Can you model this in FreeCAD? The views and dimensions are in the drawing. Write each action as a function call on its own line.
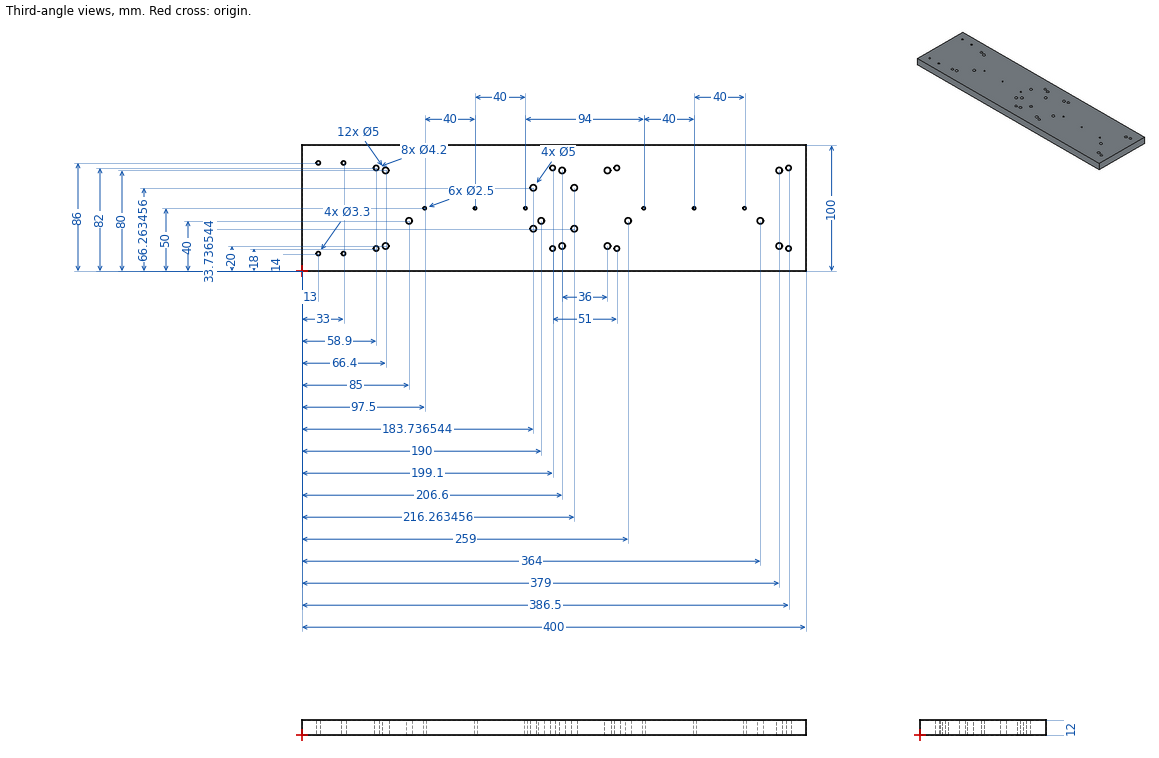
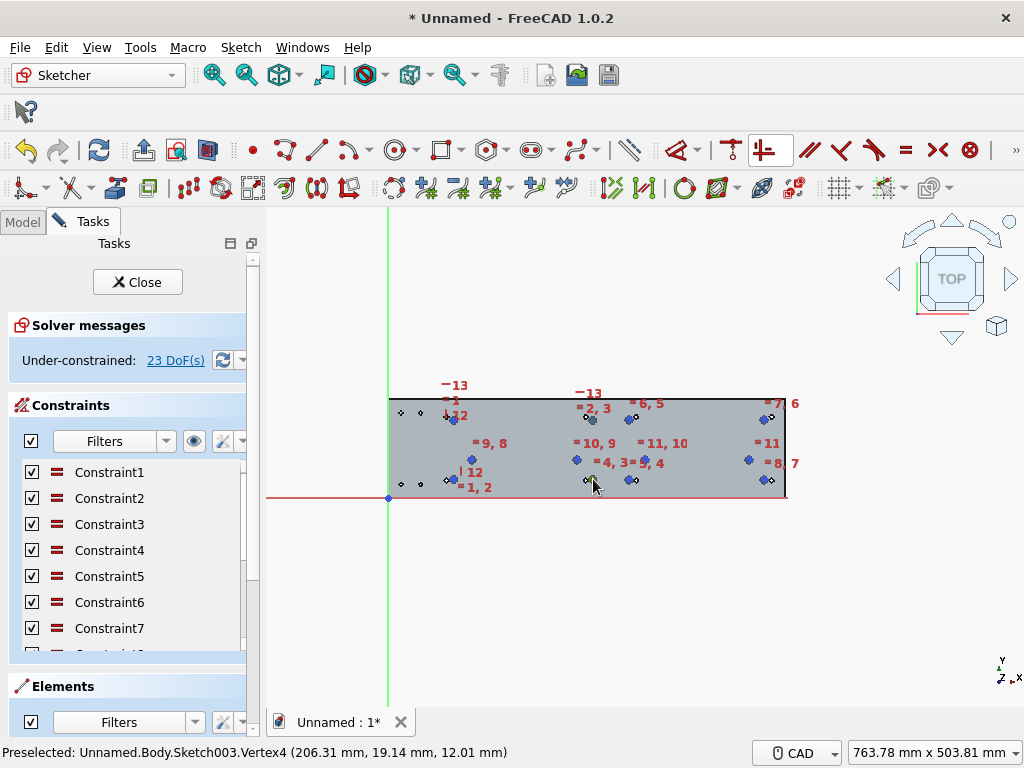
click(788, 150)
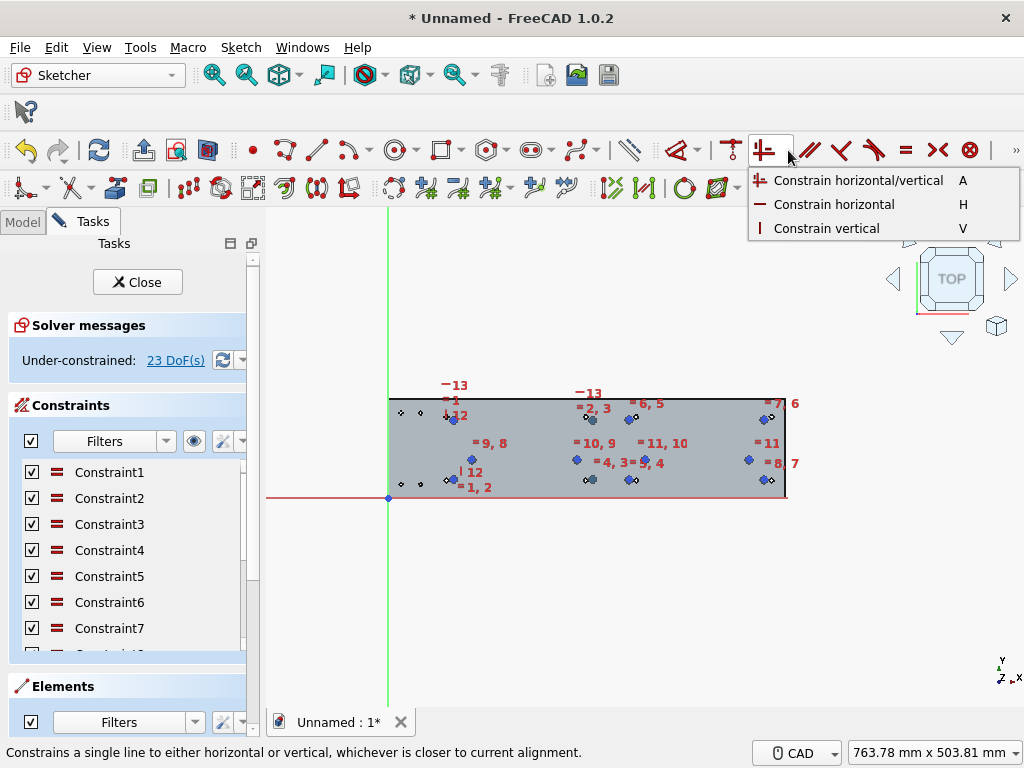
click(884, 228)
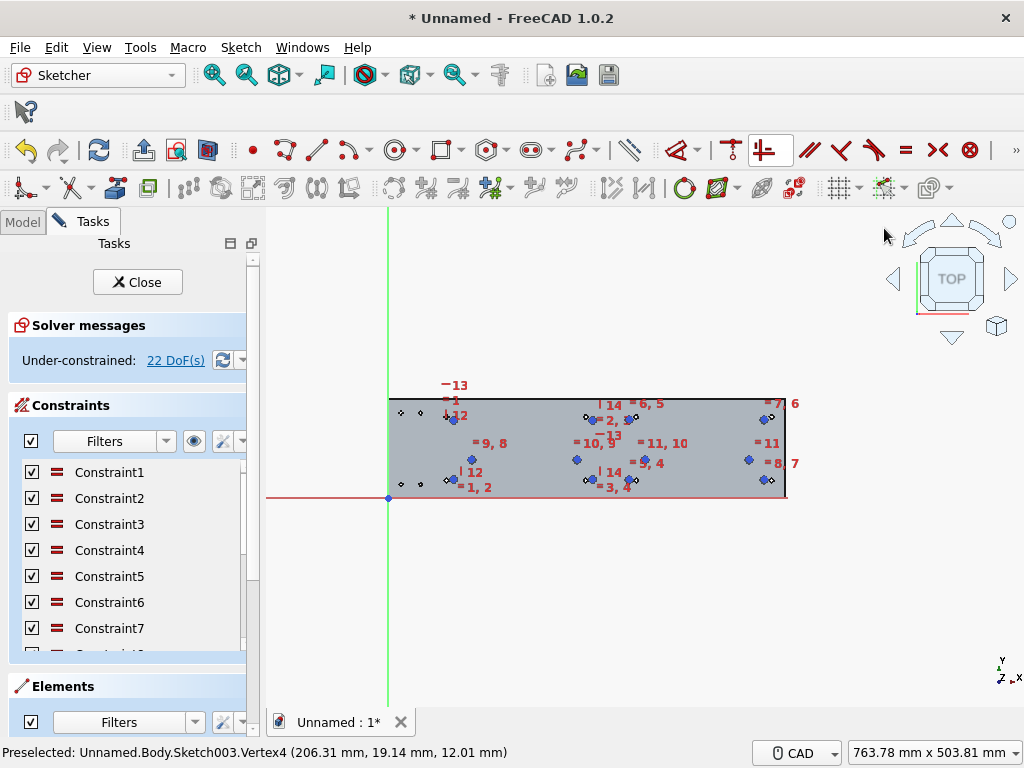
click(454, 479)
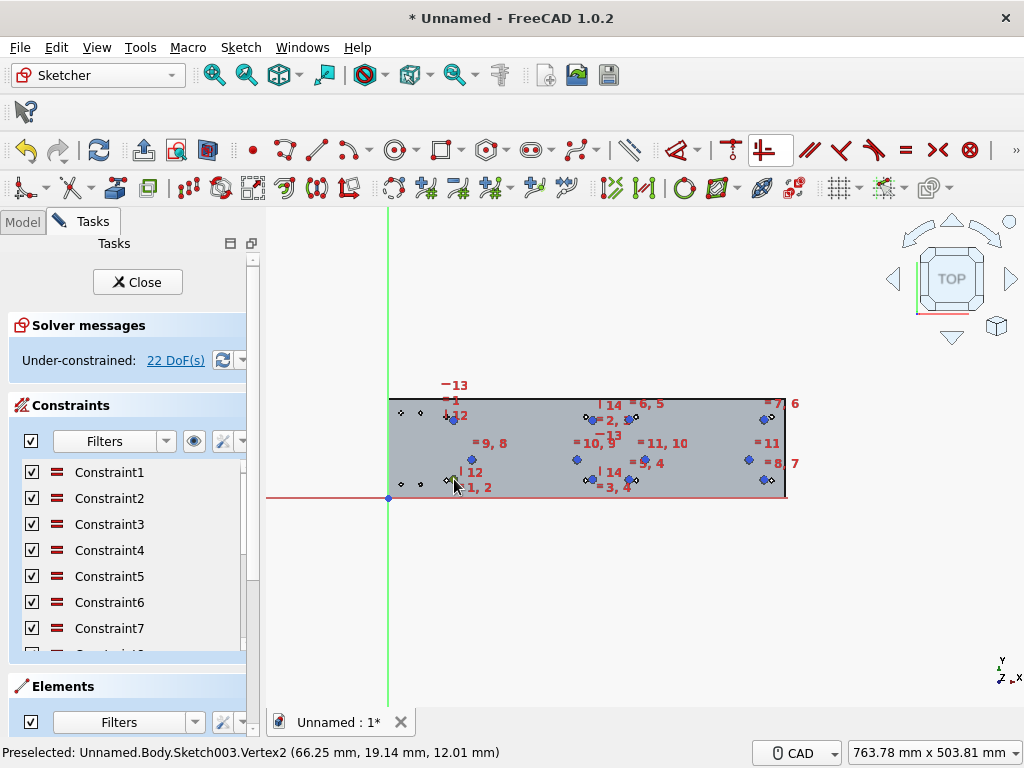
click(593, 479)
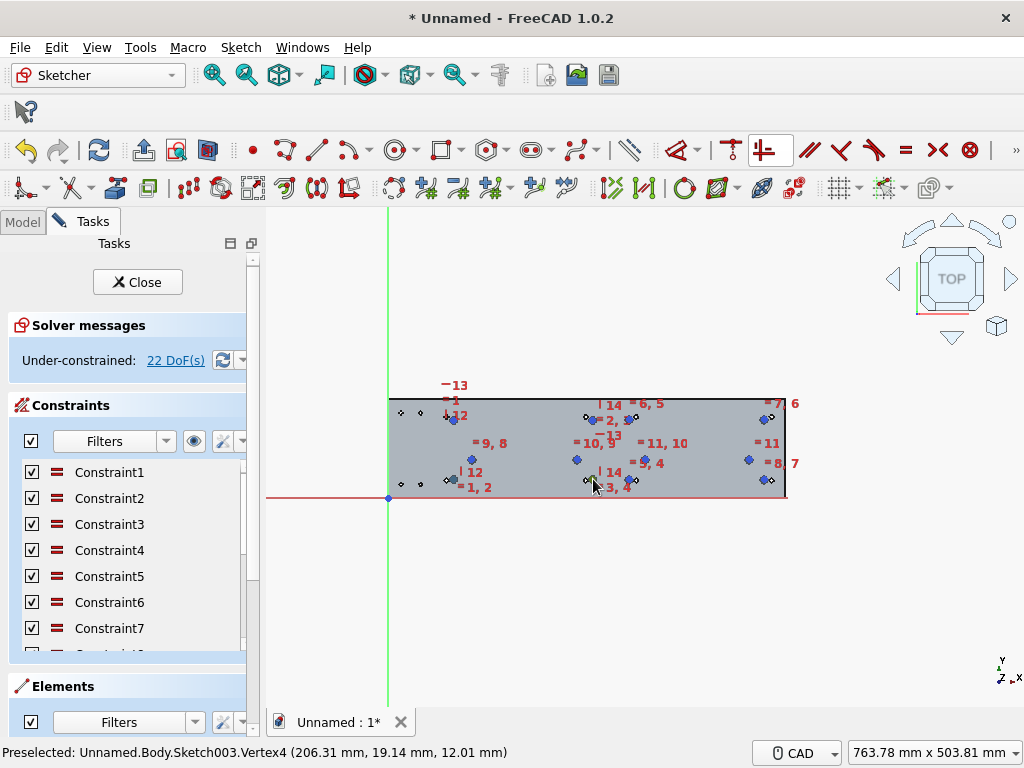
click(788, 150)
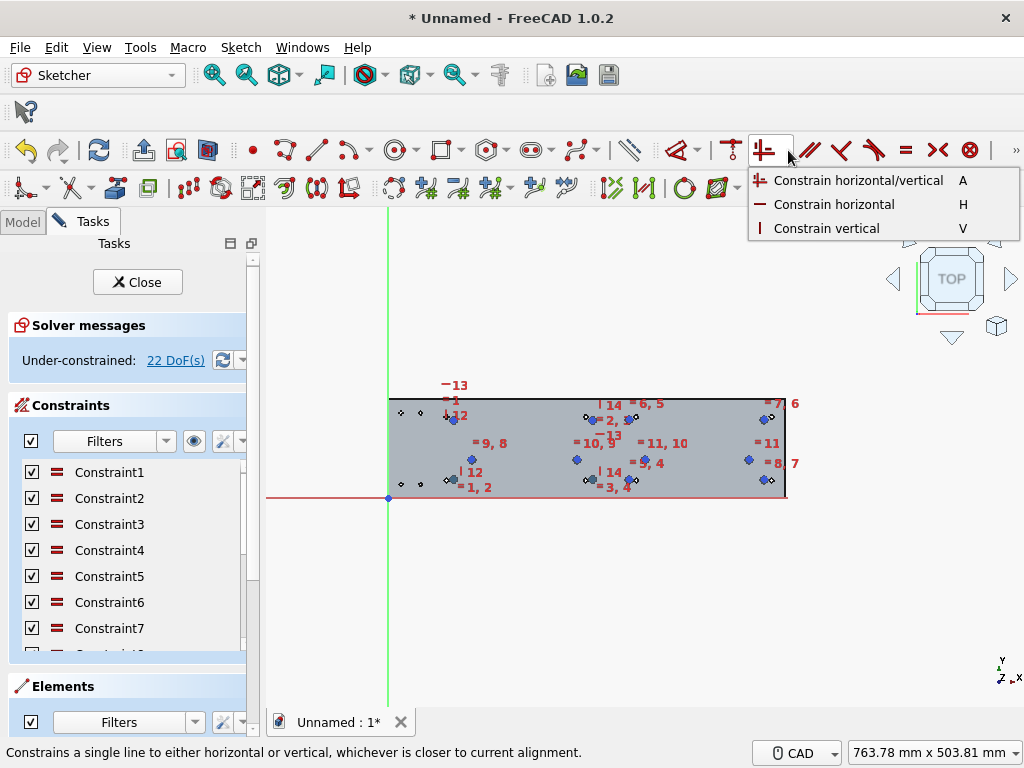
click(884, 204)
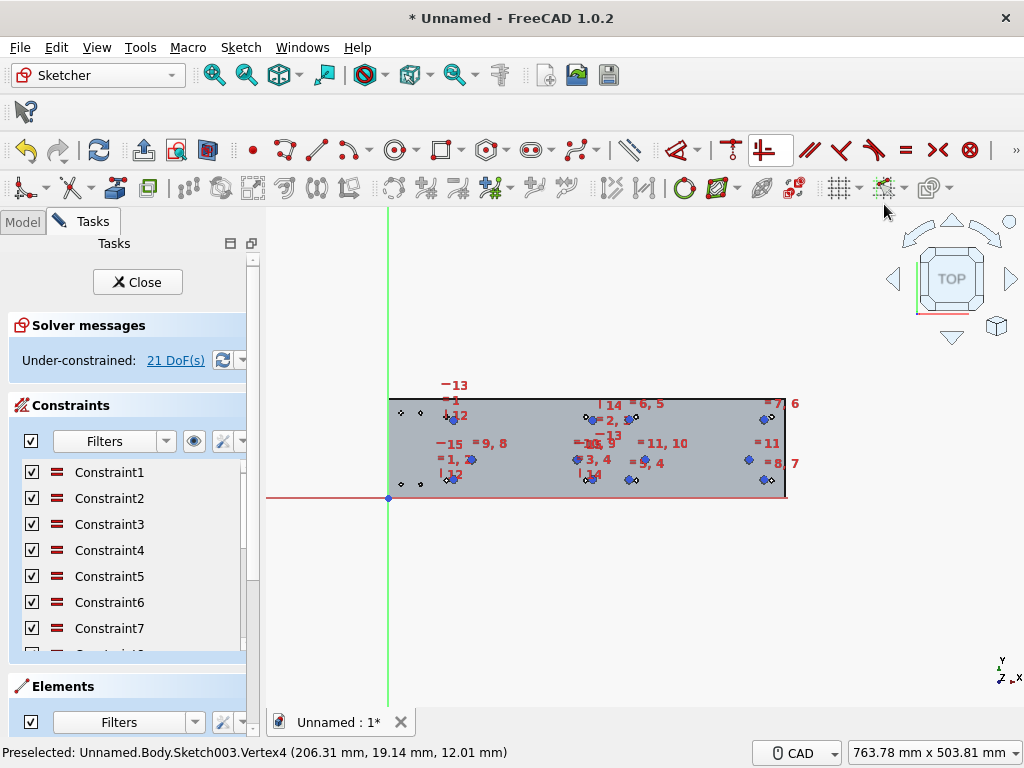
click(591, 481)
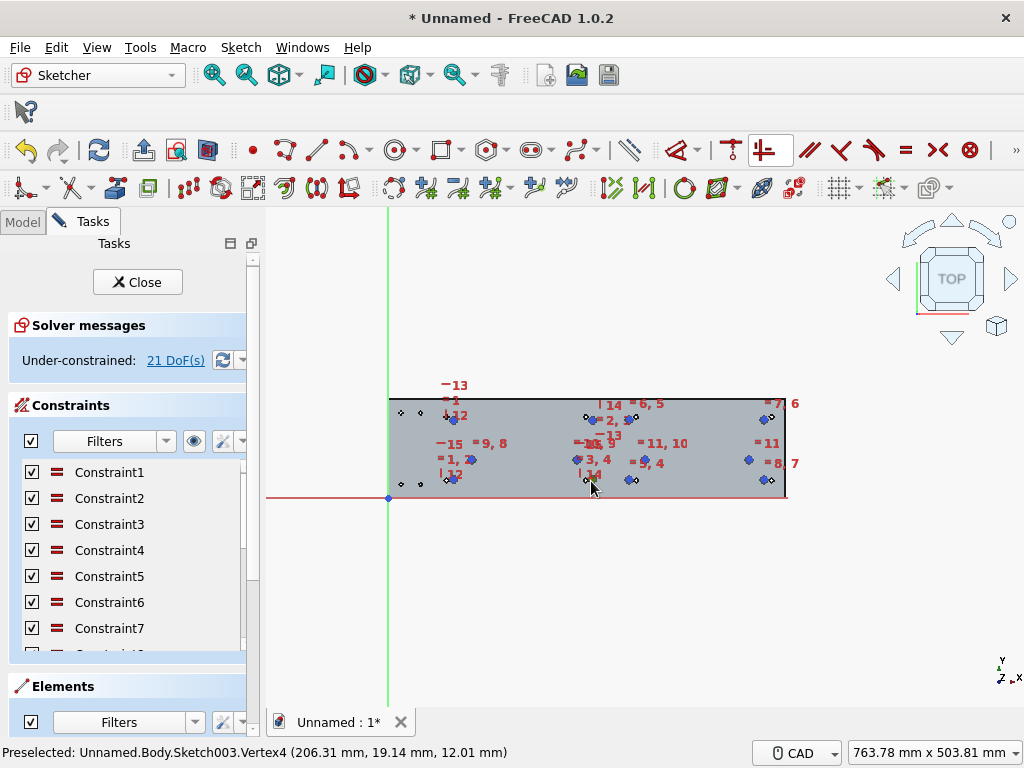
click(629, 480)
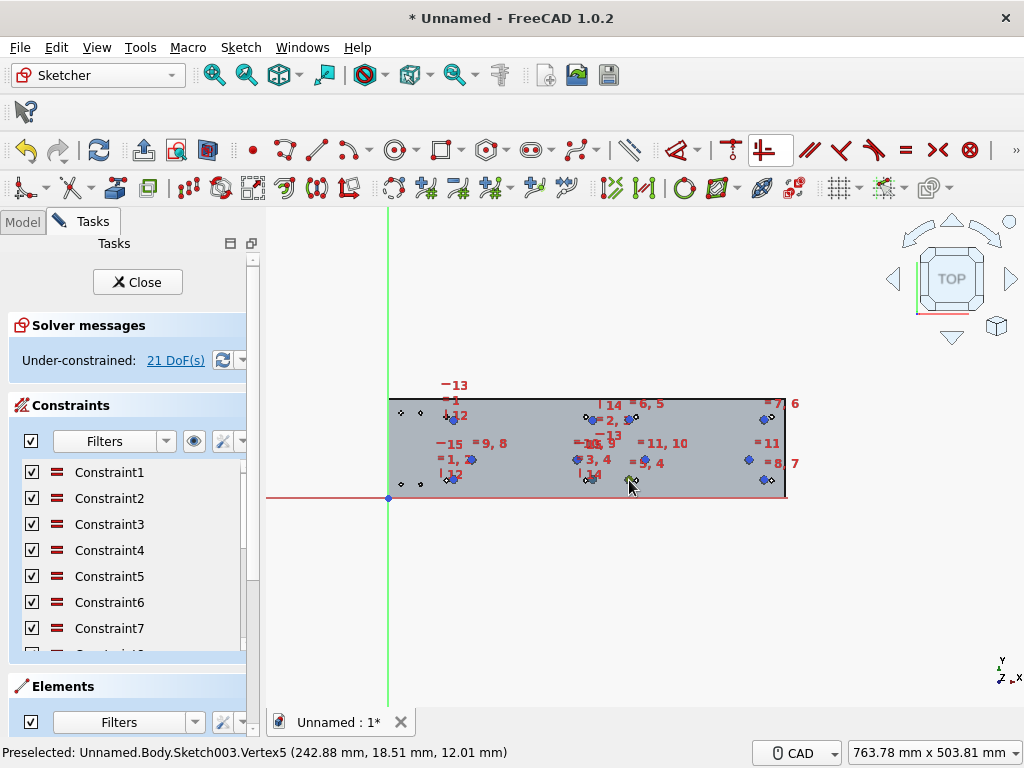
click(788, 150)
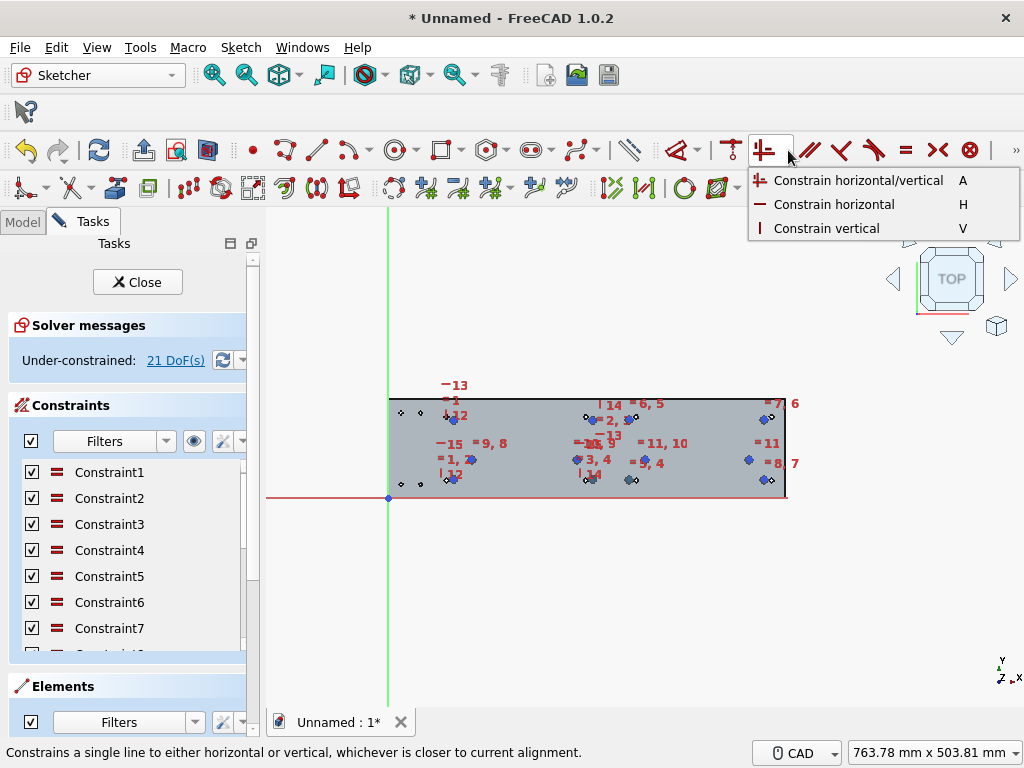
click(884, 204)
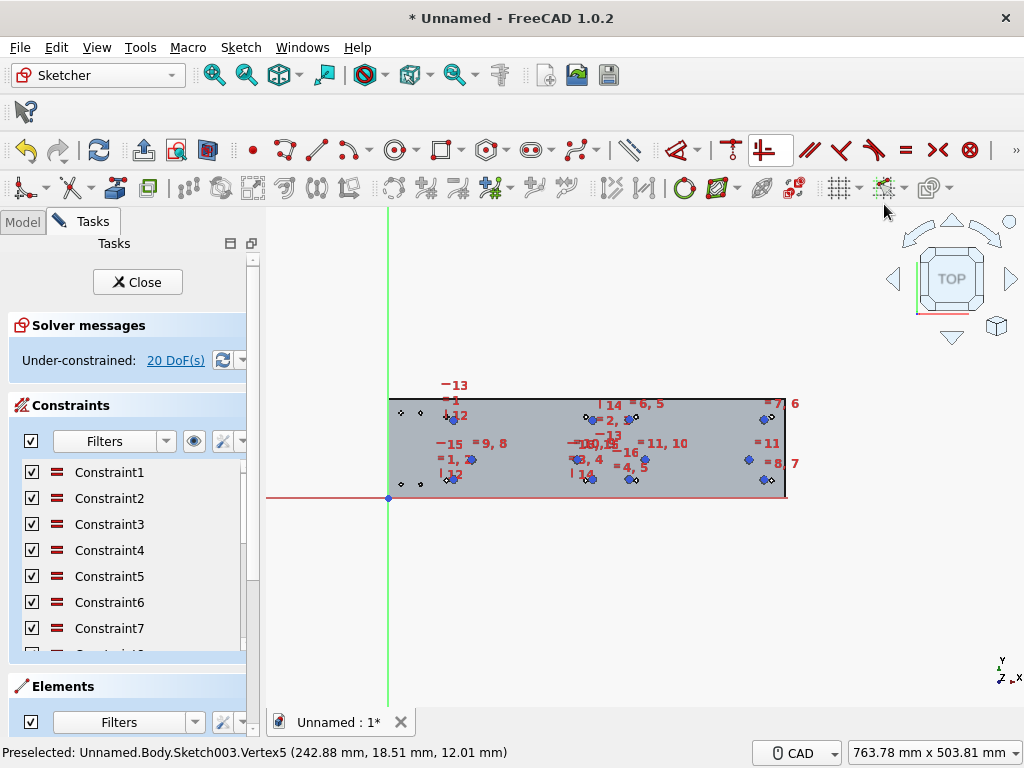
click(629, 479)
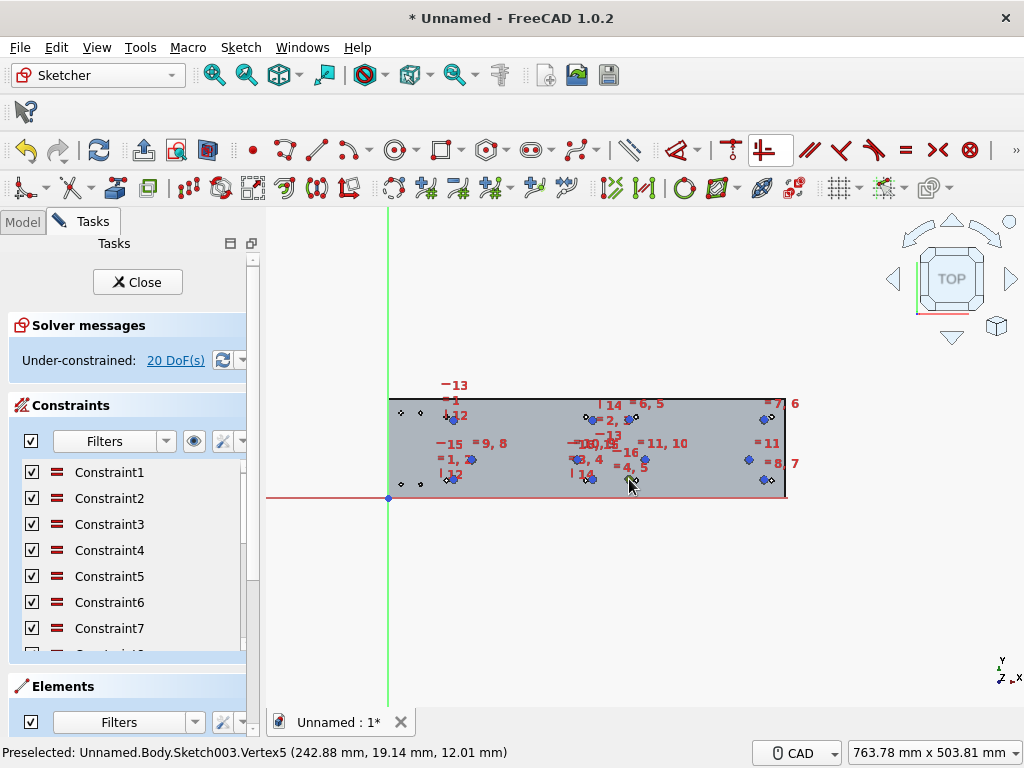
click(629, 420)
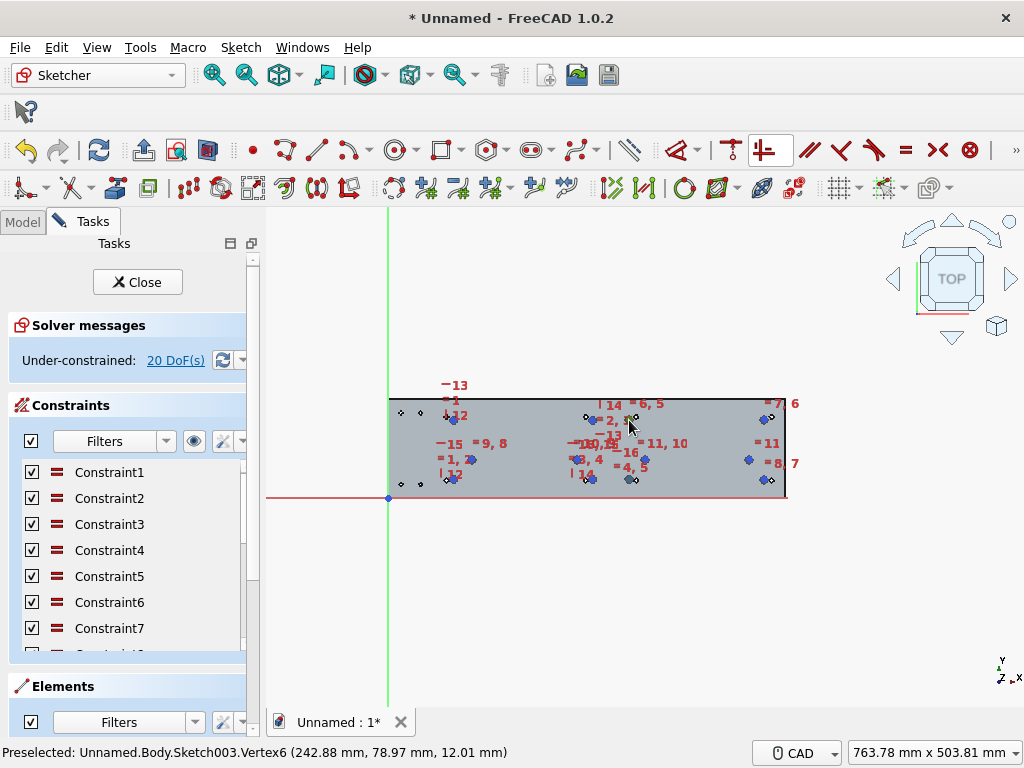
click(788, 150)